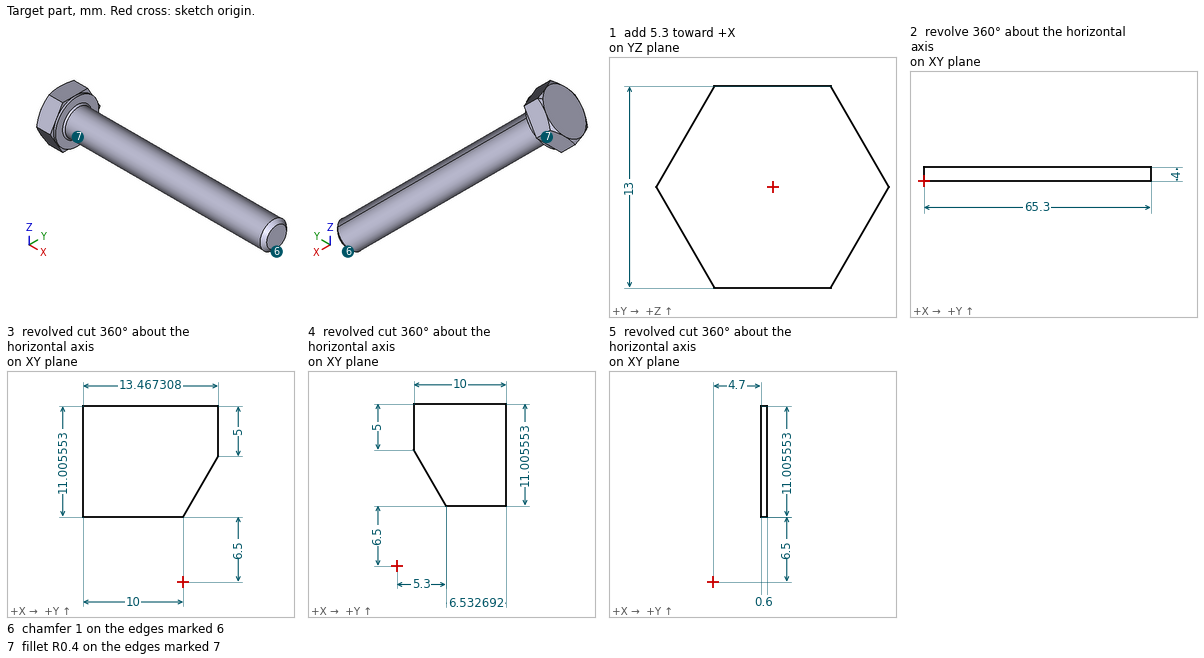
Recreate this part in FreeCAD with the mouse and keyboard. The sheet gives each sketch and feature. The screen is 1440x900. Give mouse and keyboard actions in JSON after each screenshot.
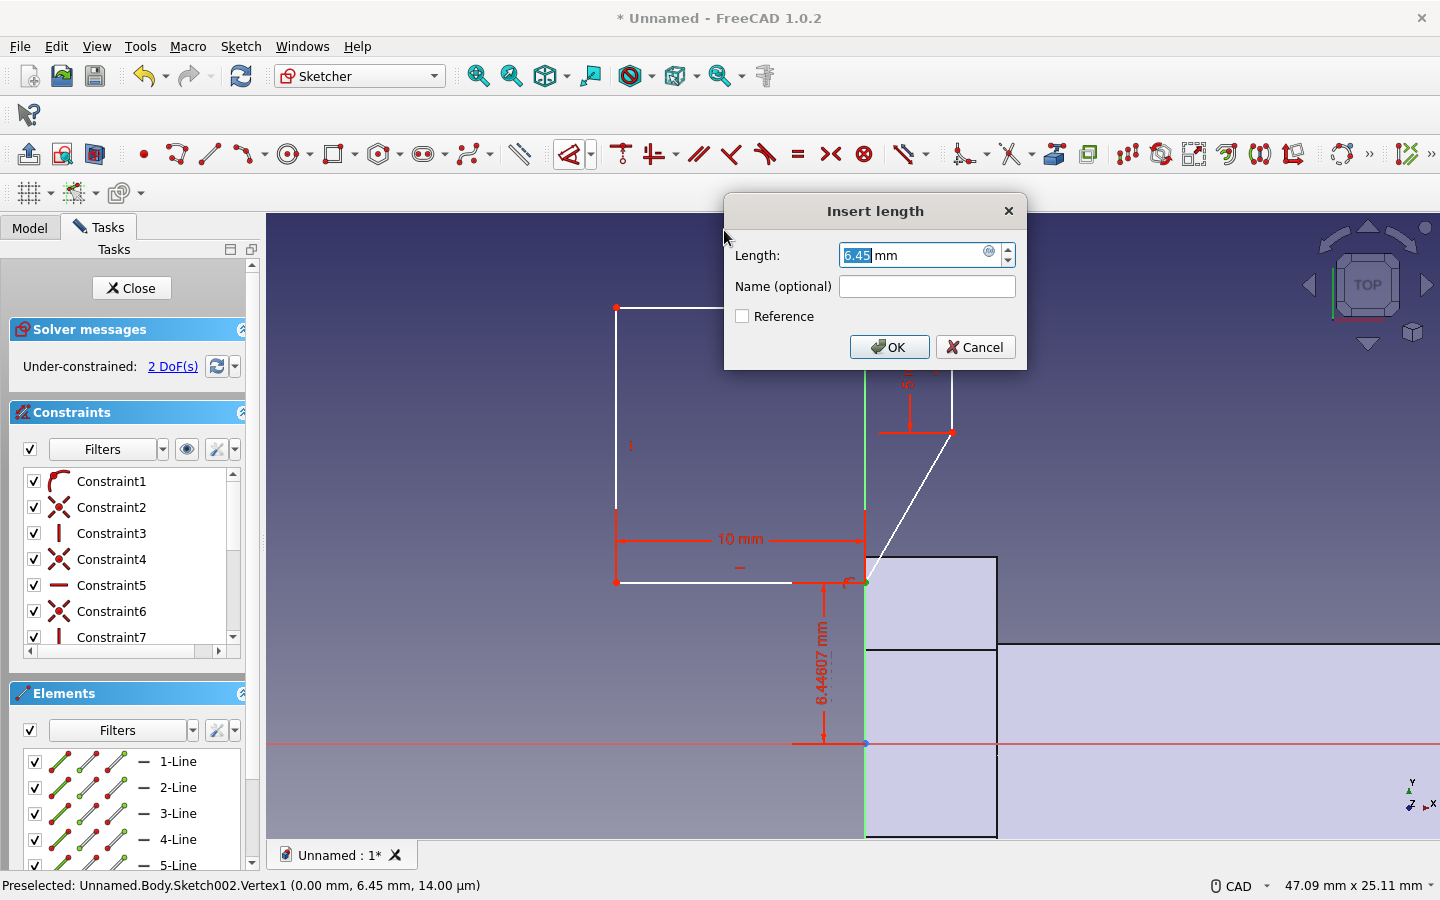
{"action": "type", "text": "6.5"}
{"action": "key", "text": "Return"}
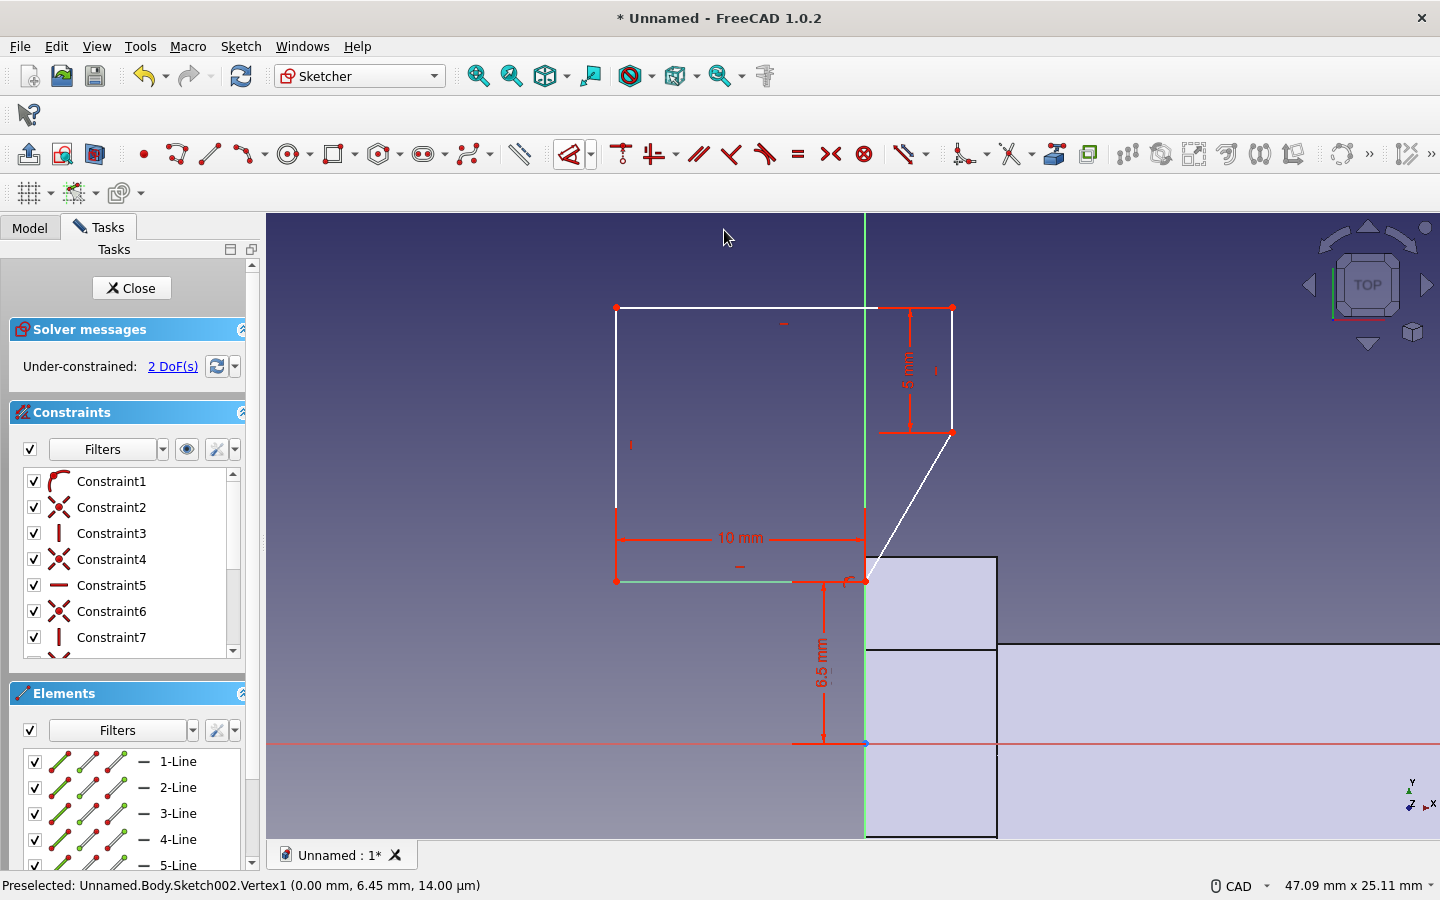
{"action": "left_click", "coordinate": [851, 308]}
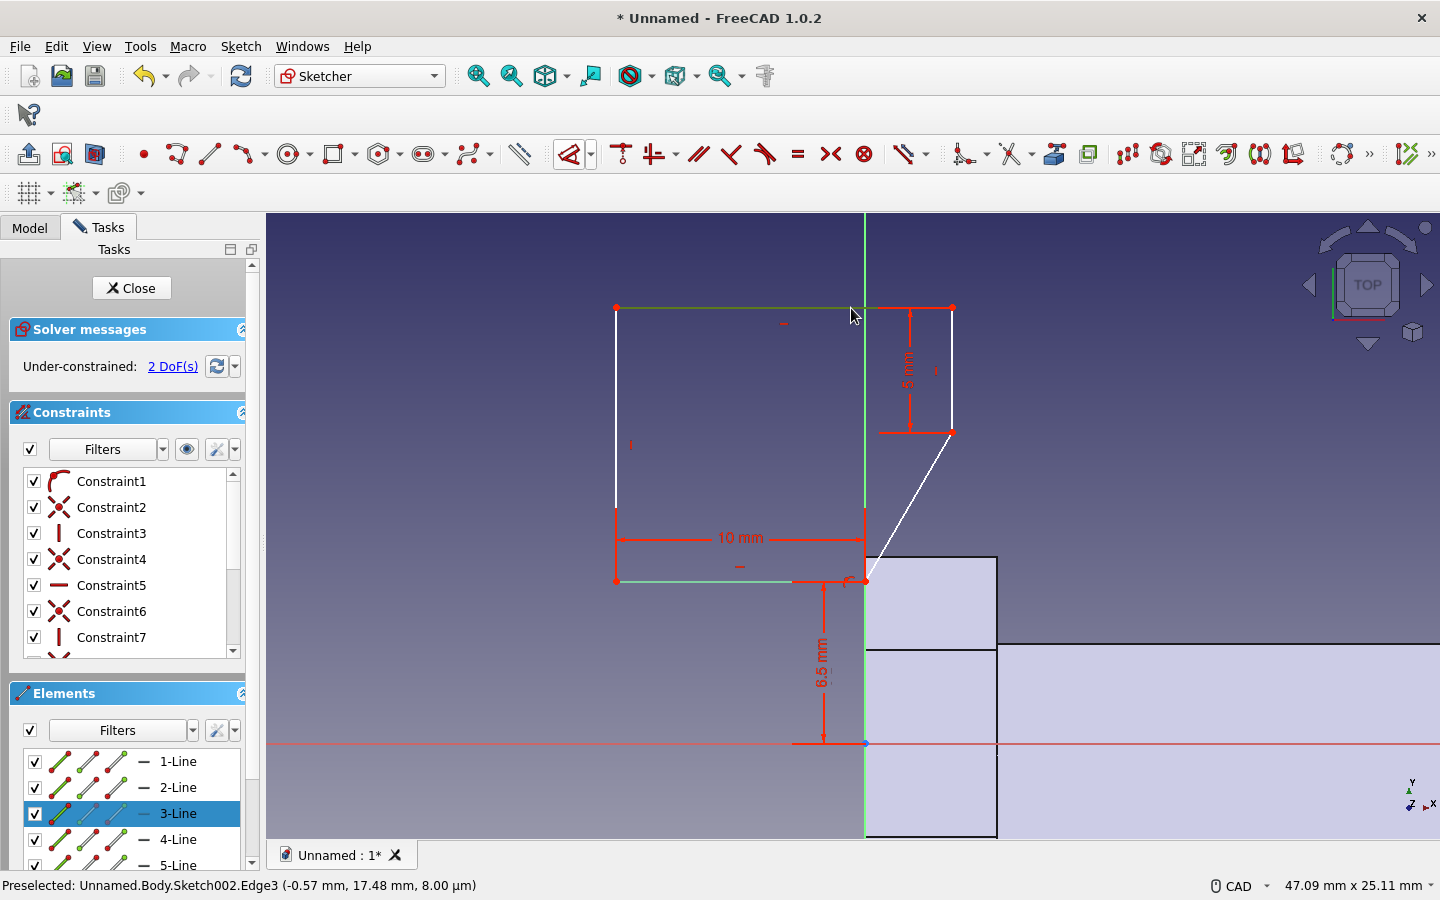
{"action": "left_click", "coordinate": [590, 154]}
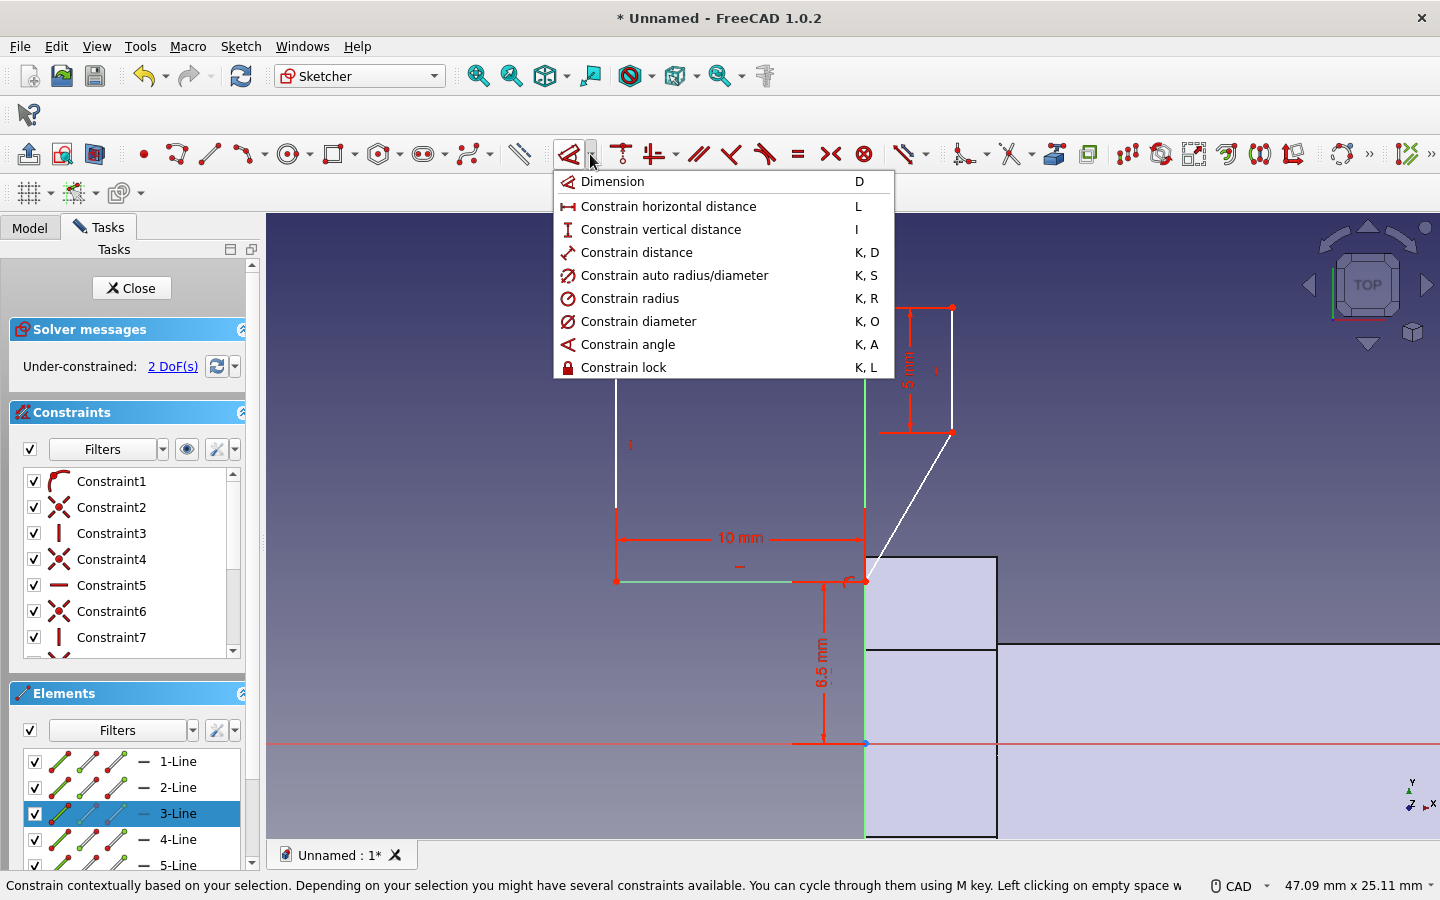
{"action": "left_click", "coordinate": [724, 206]}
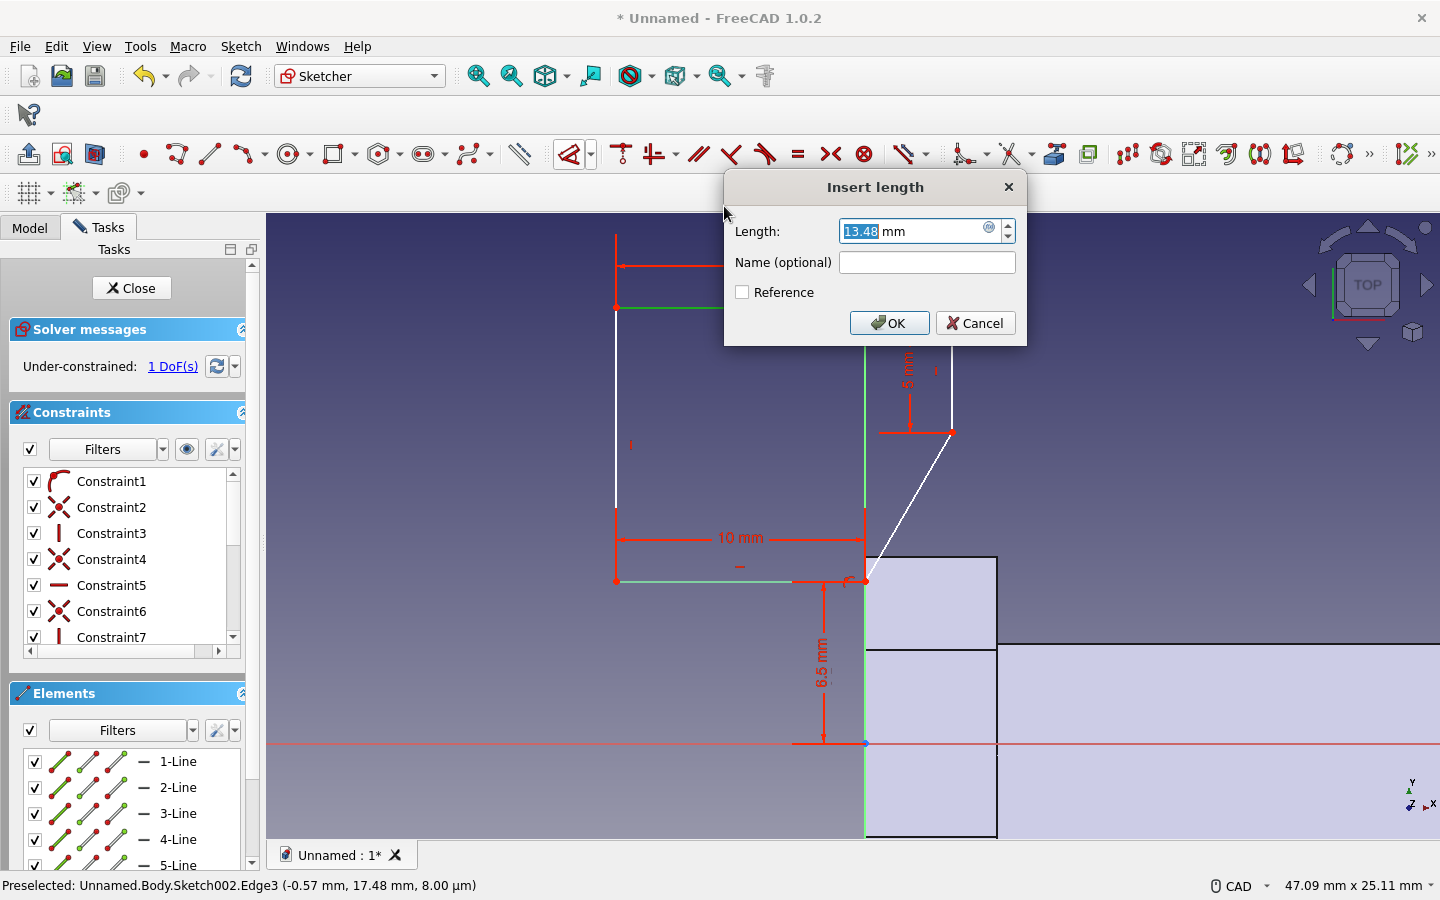
{"action": "type", "text": "13.467308"}
{"action": "key", "text": "Return"}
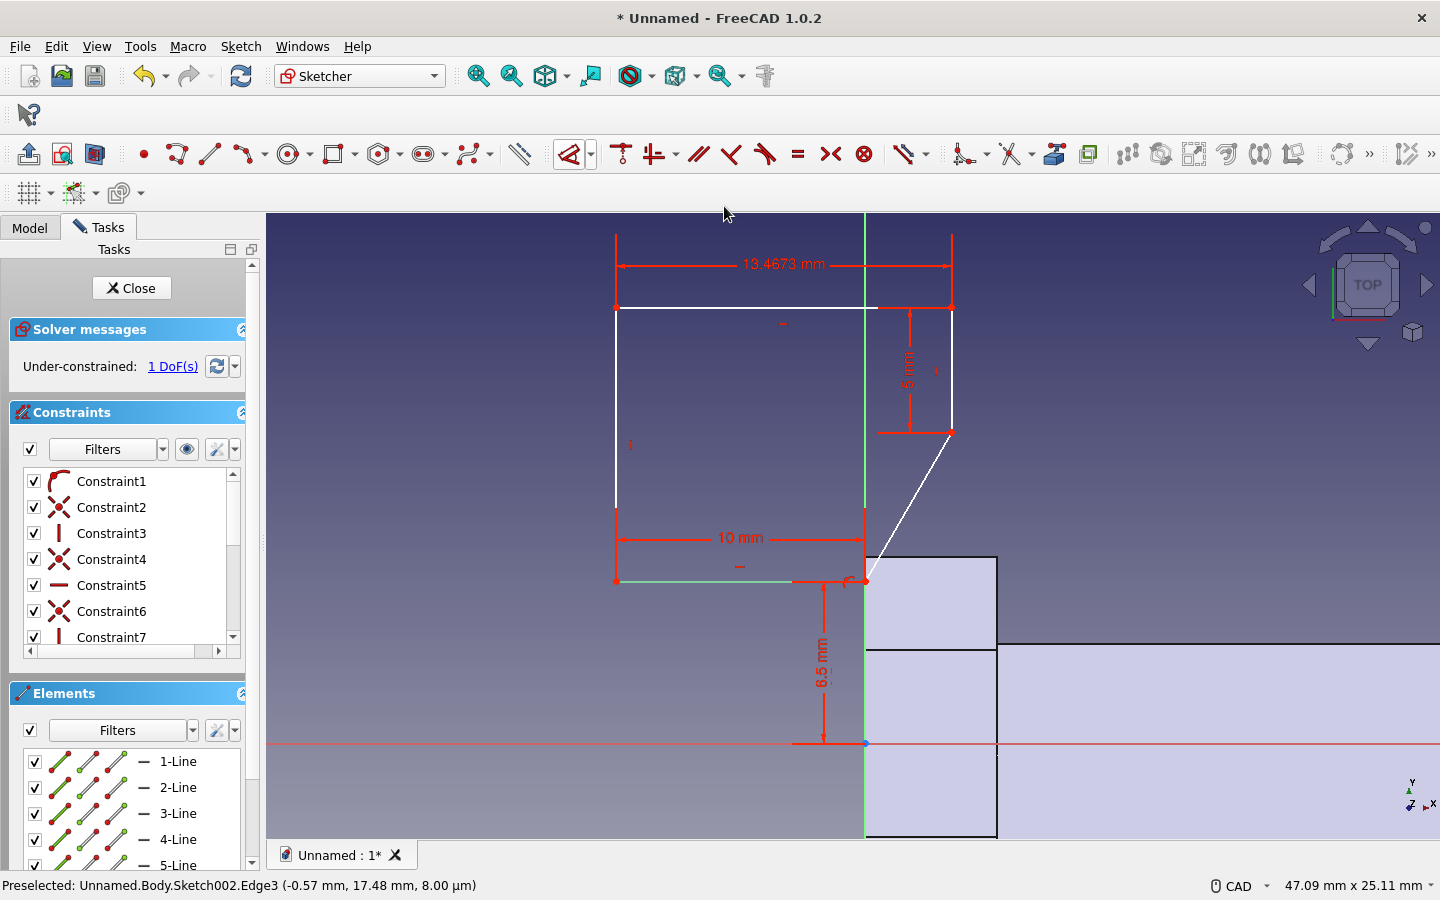
{"action": "left_click", "coordinate": [616, 390]}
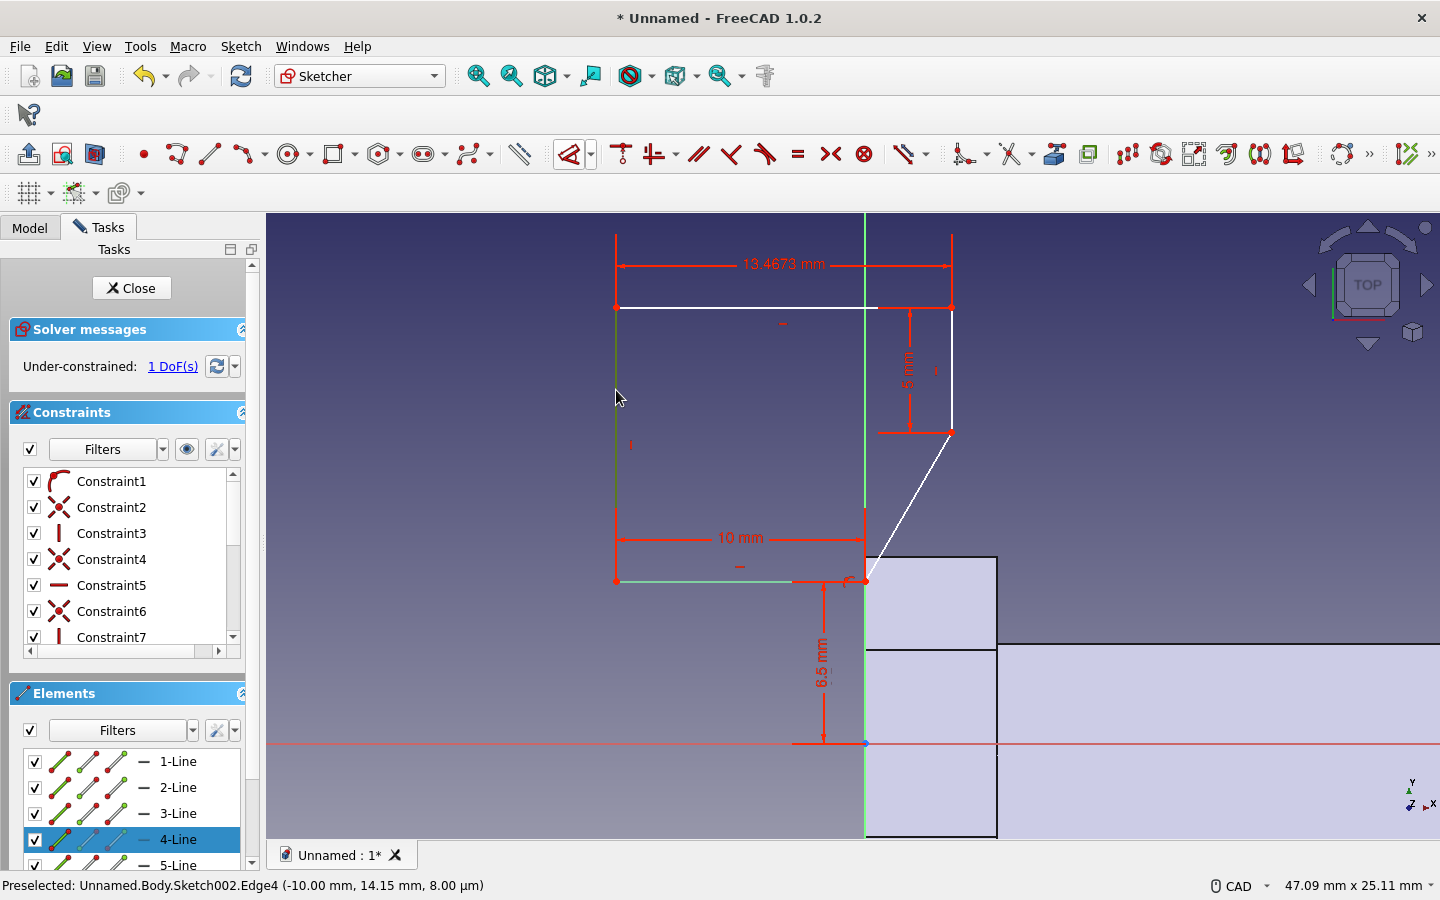
{"action": "left_click", "coordinate": [590, 154]}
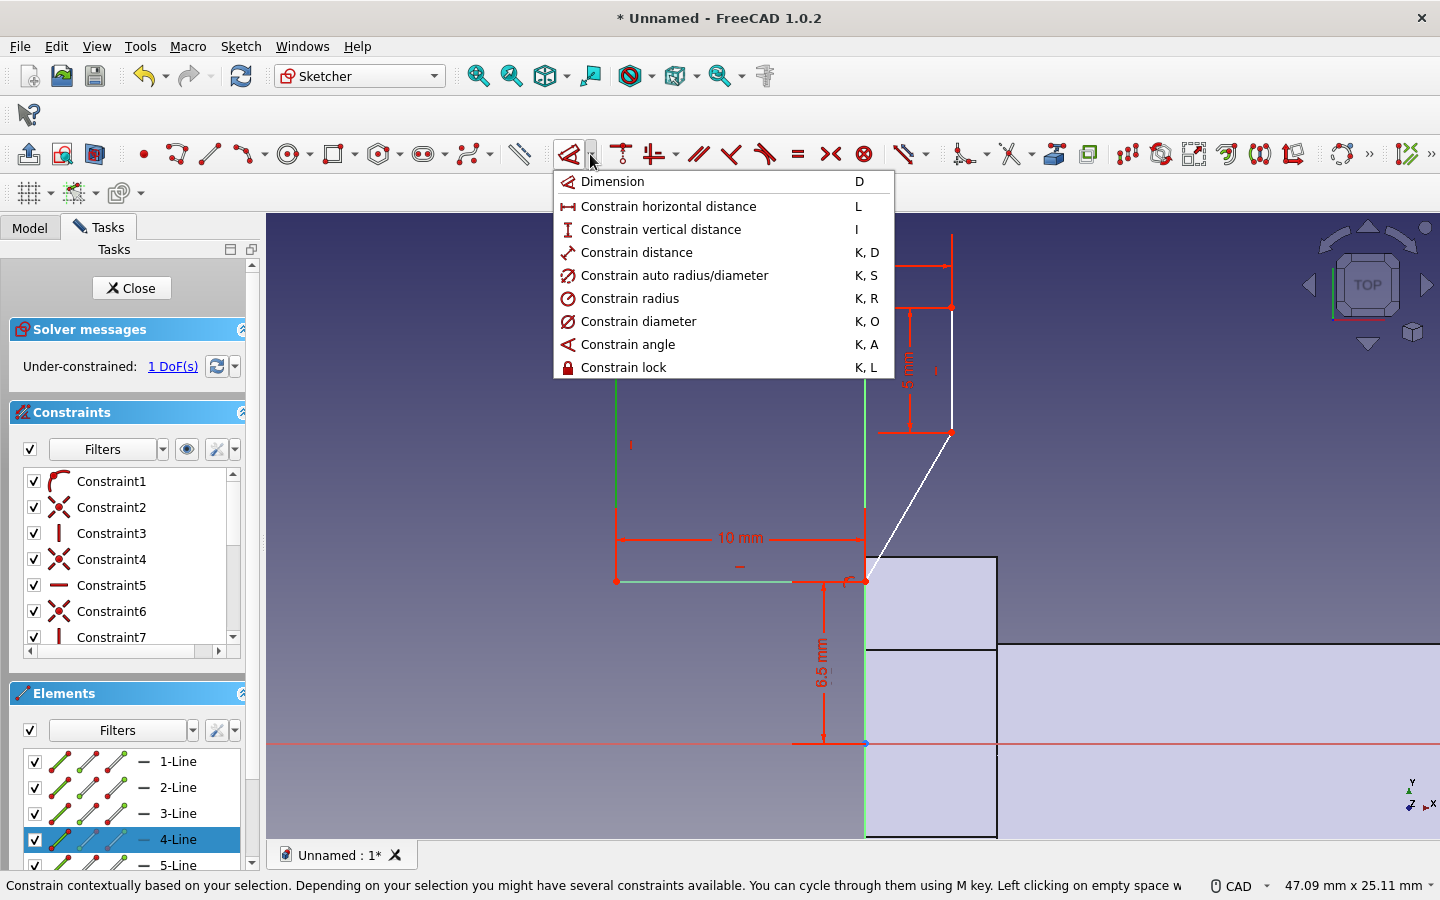
{"action": "left_click", "coordinate": [724, 230]}